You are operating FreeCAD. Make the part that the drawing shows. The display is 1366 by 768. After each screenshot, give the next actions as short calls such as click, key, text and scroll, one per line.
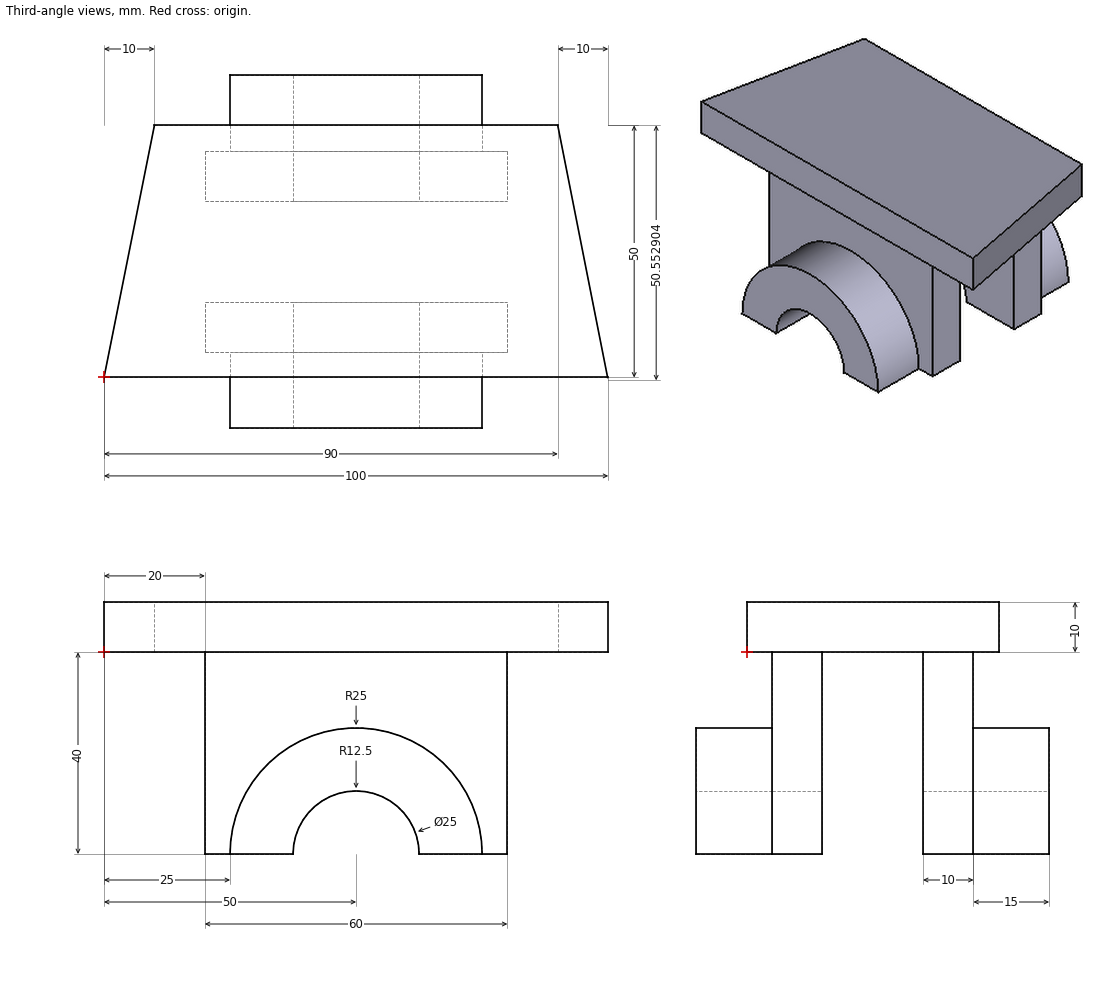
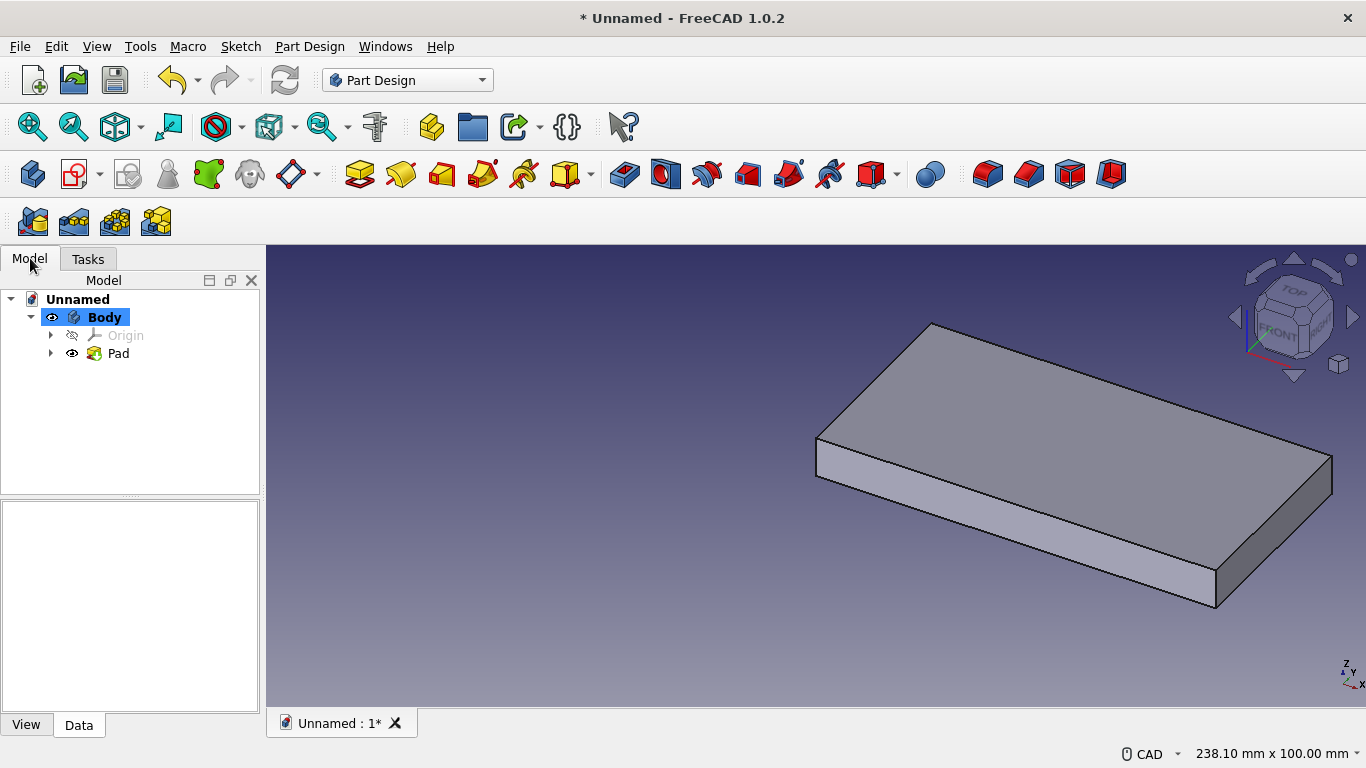
click(51, 335)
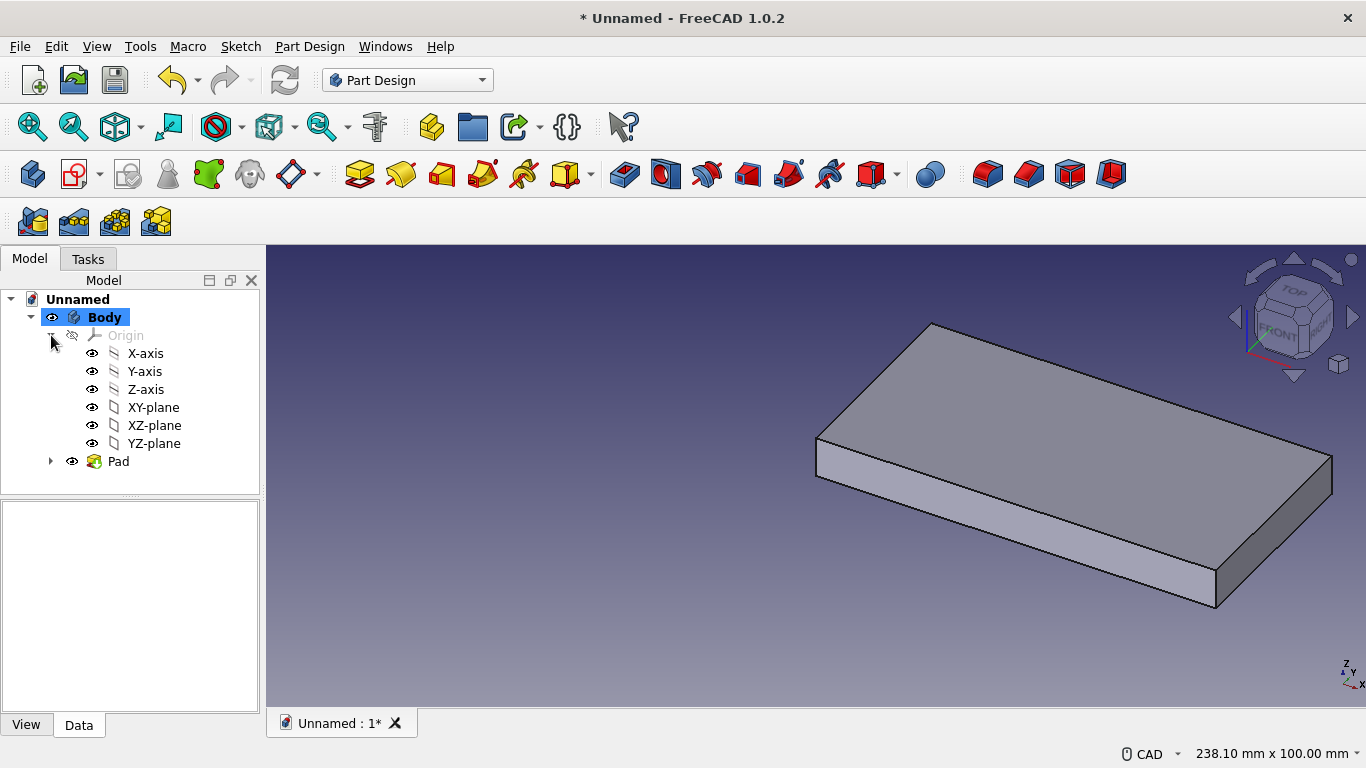
click(137, 425)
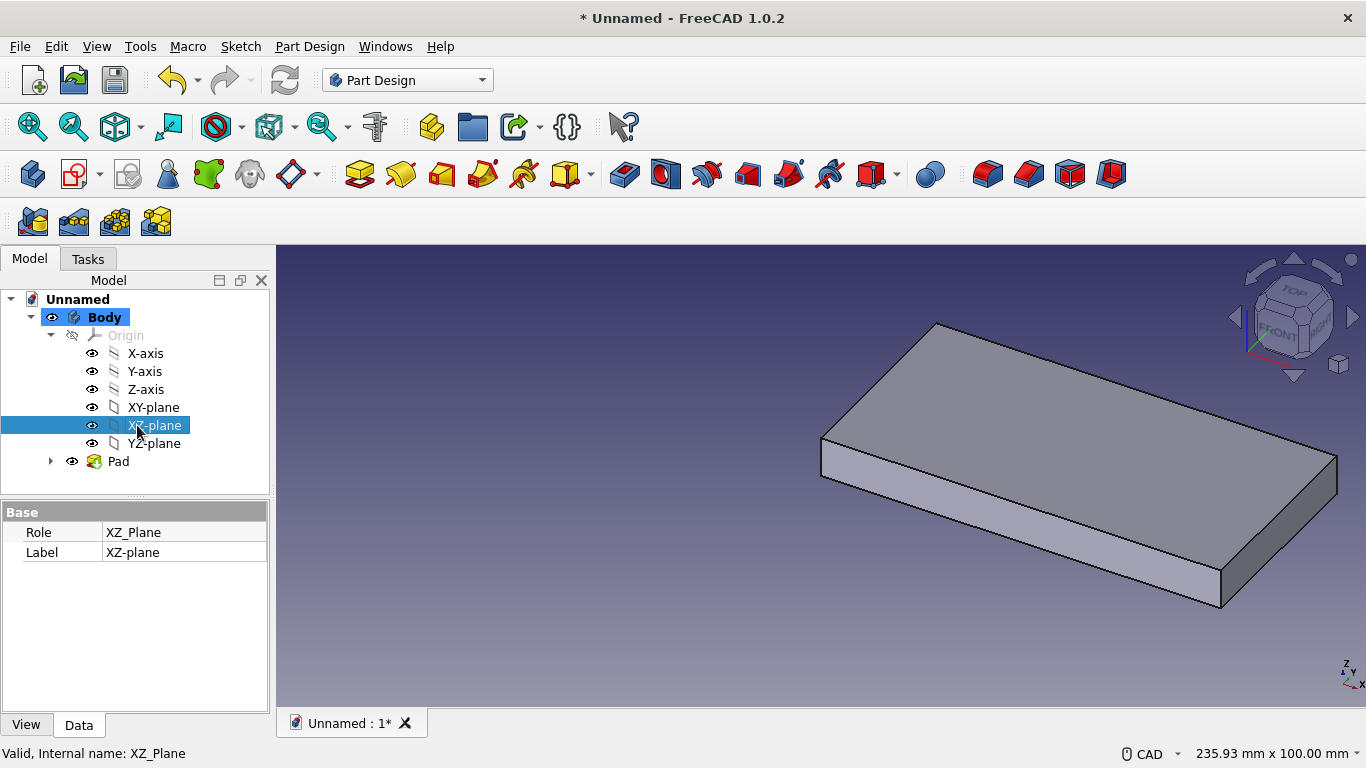
click(290, 174)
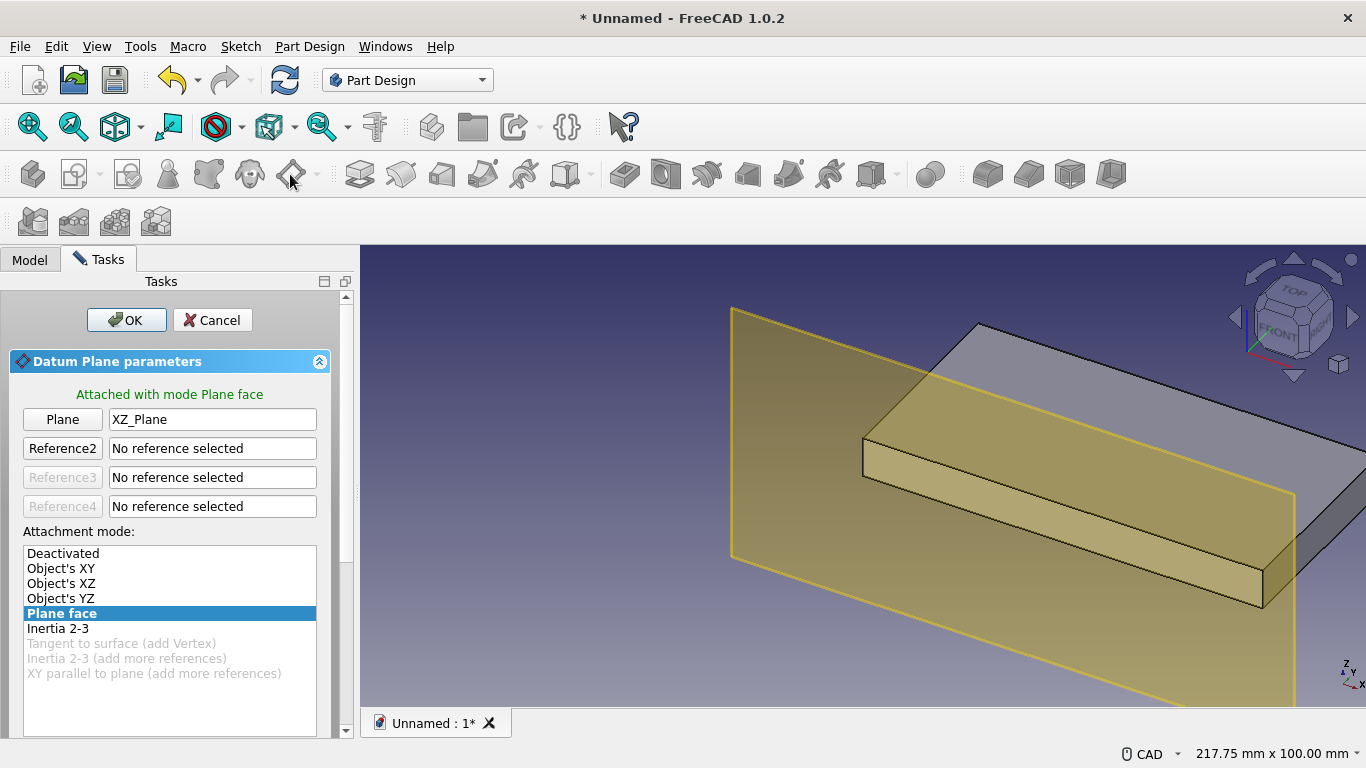
scroll(346, 514, down, 4)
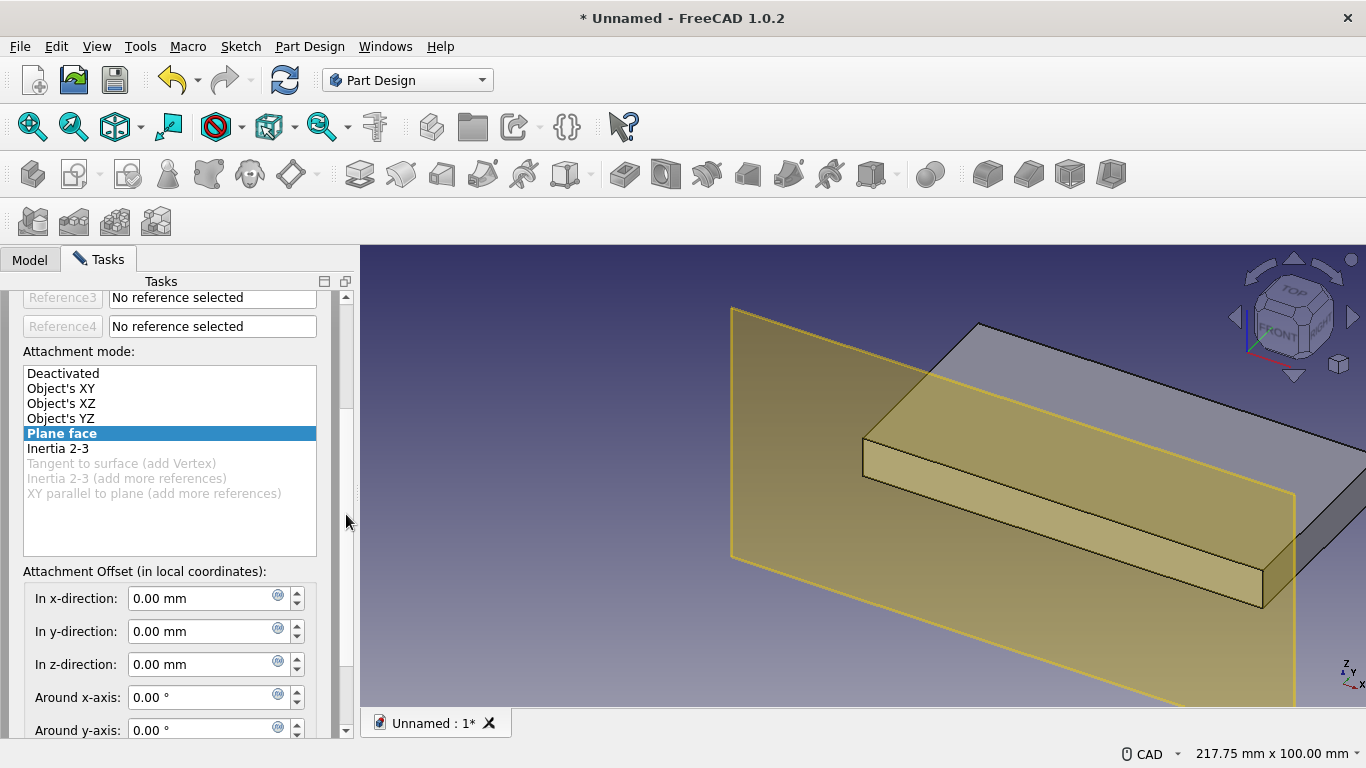
triple_click(210, 604)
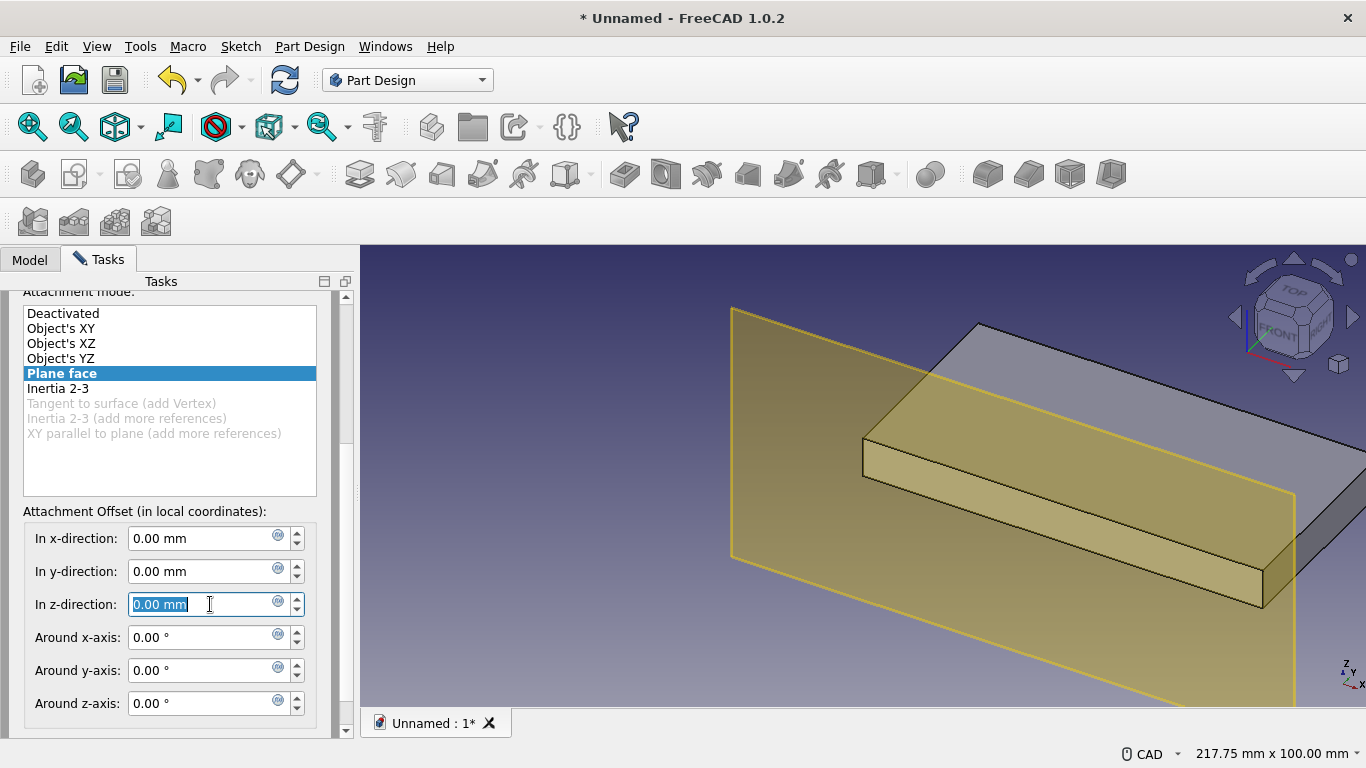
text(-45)
key(Tab)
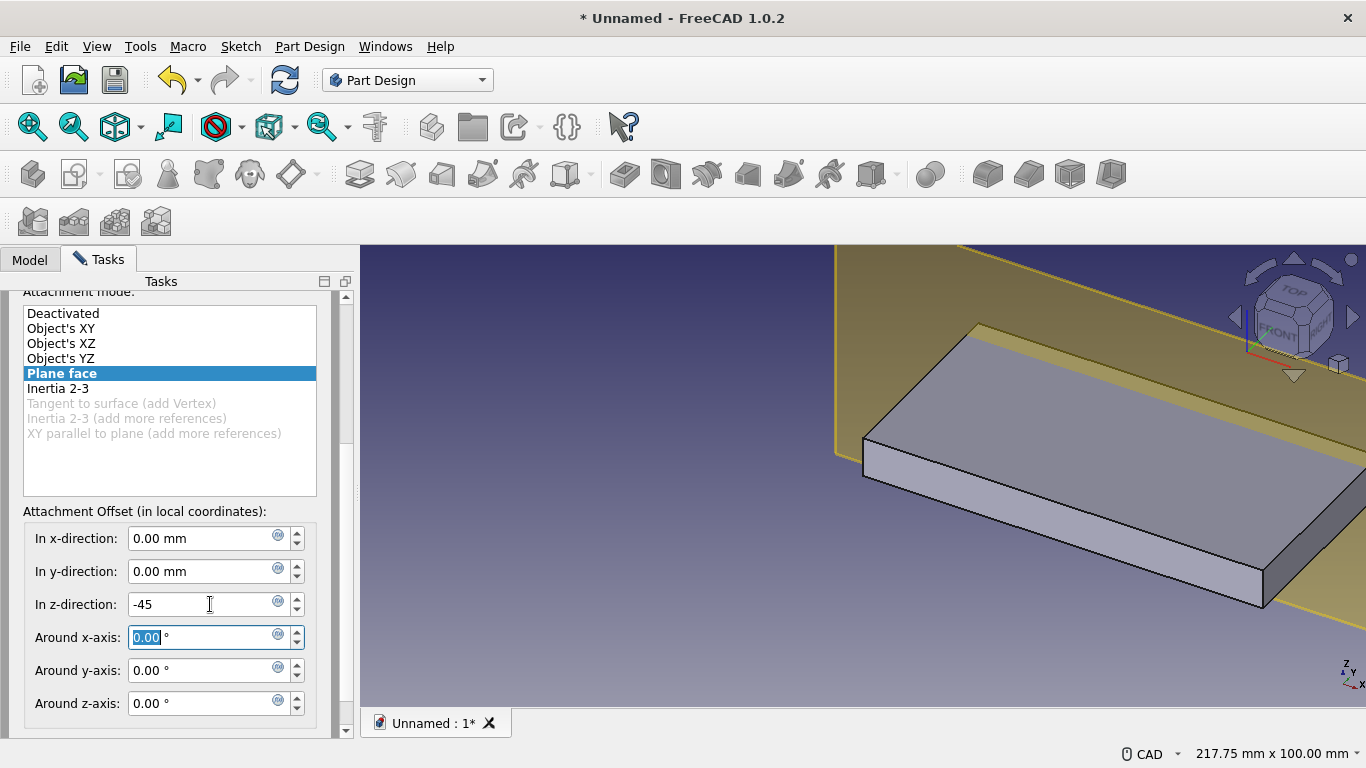
scroll(346, 514, up, 5)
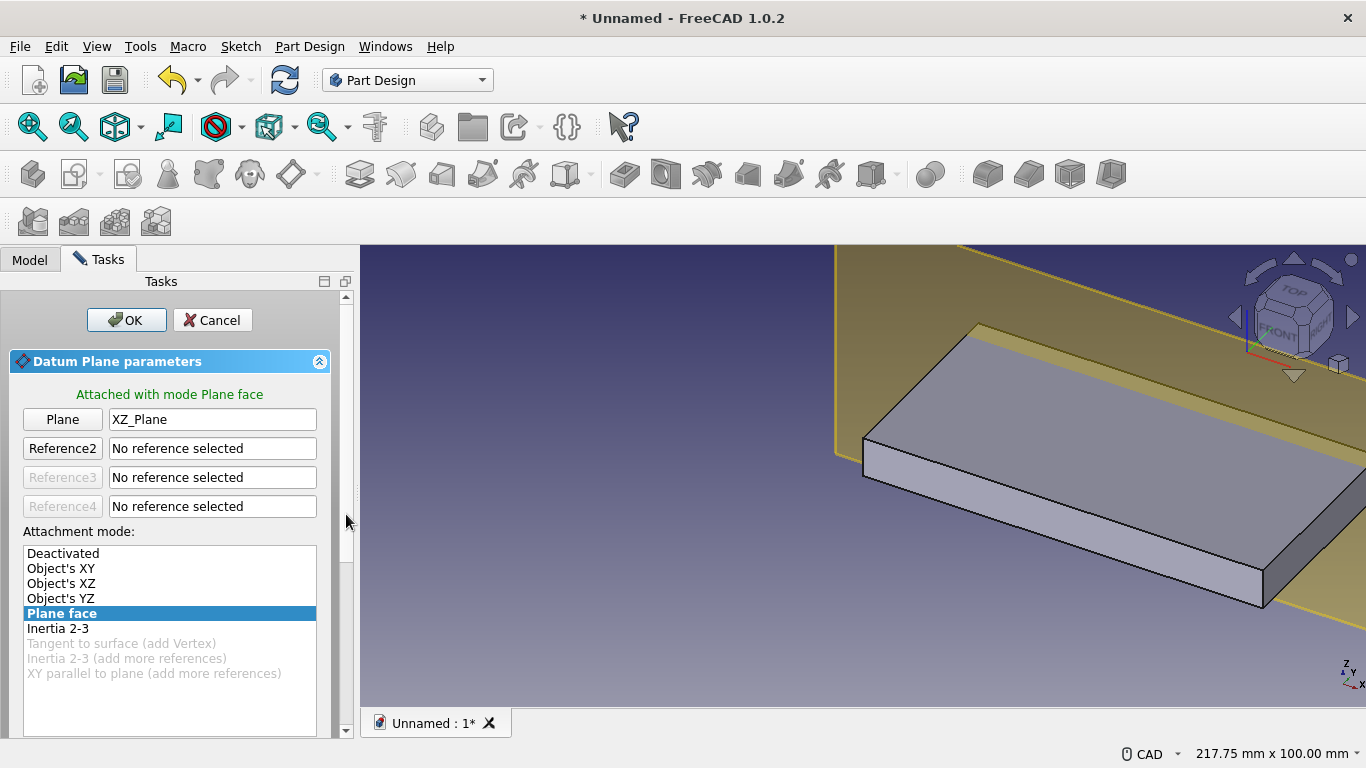
click(127, 320)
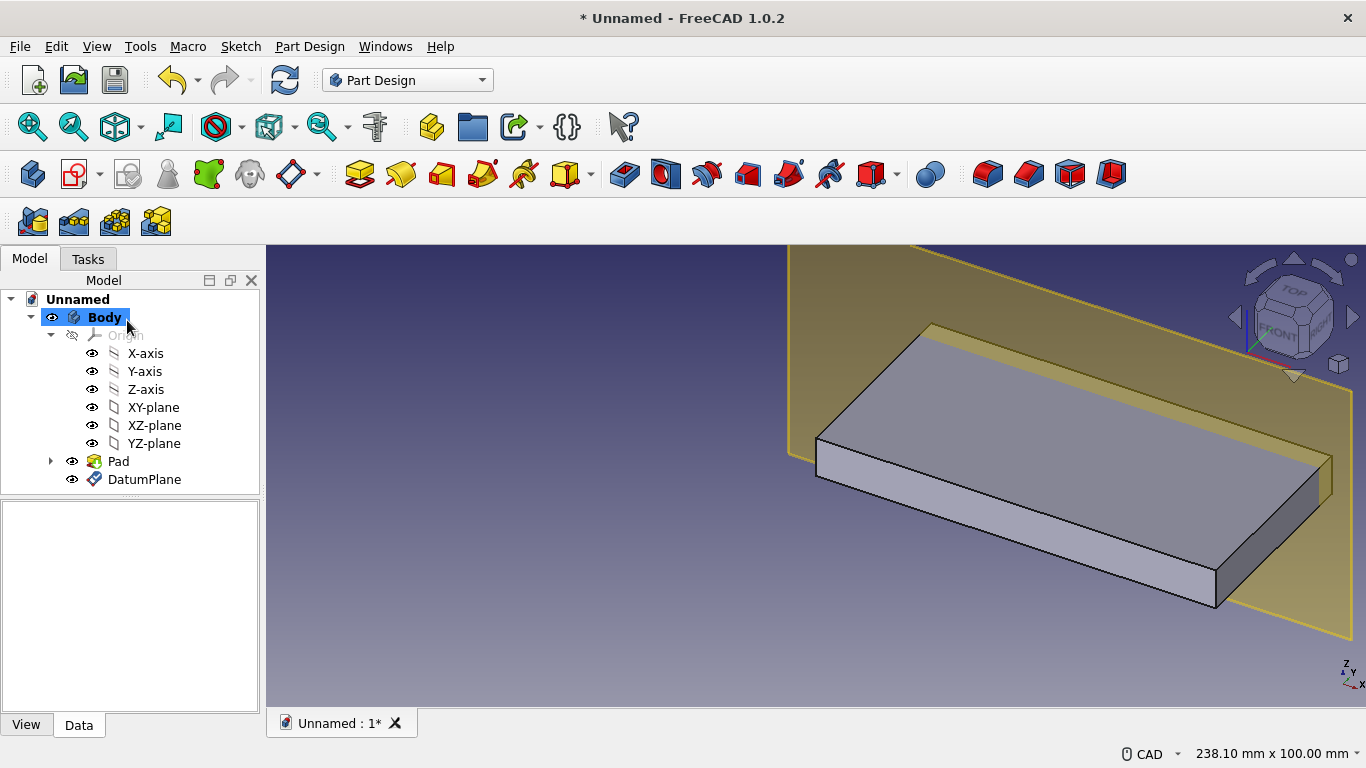
click(117, 479)